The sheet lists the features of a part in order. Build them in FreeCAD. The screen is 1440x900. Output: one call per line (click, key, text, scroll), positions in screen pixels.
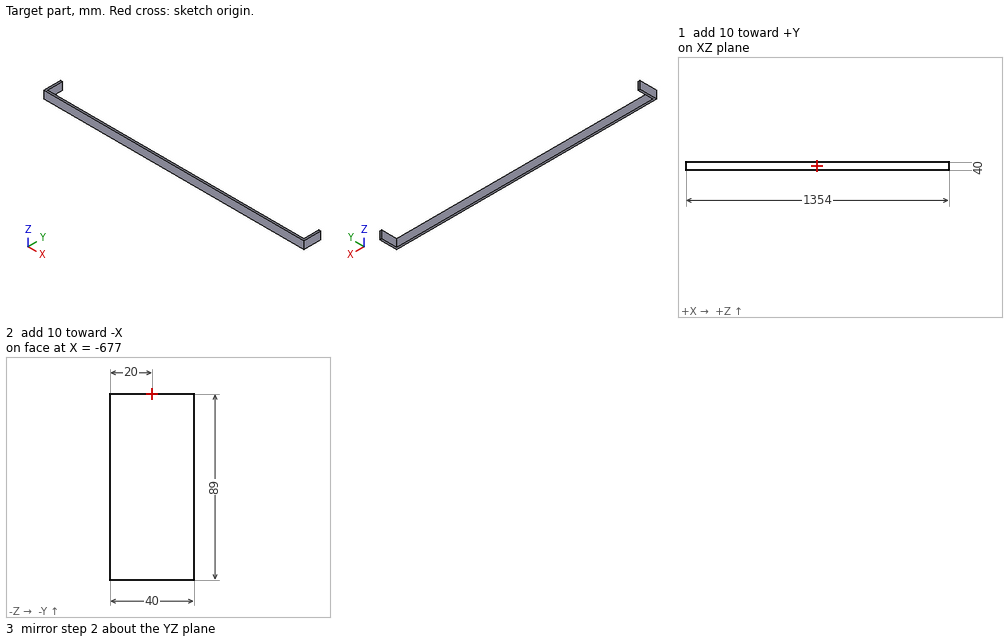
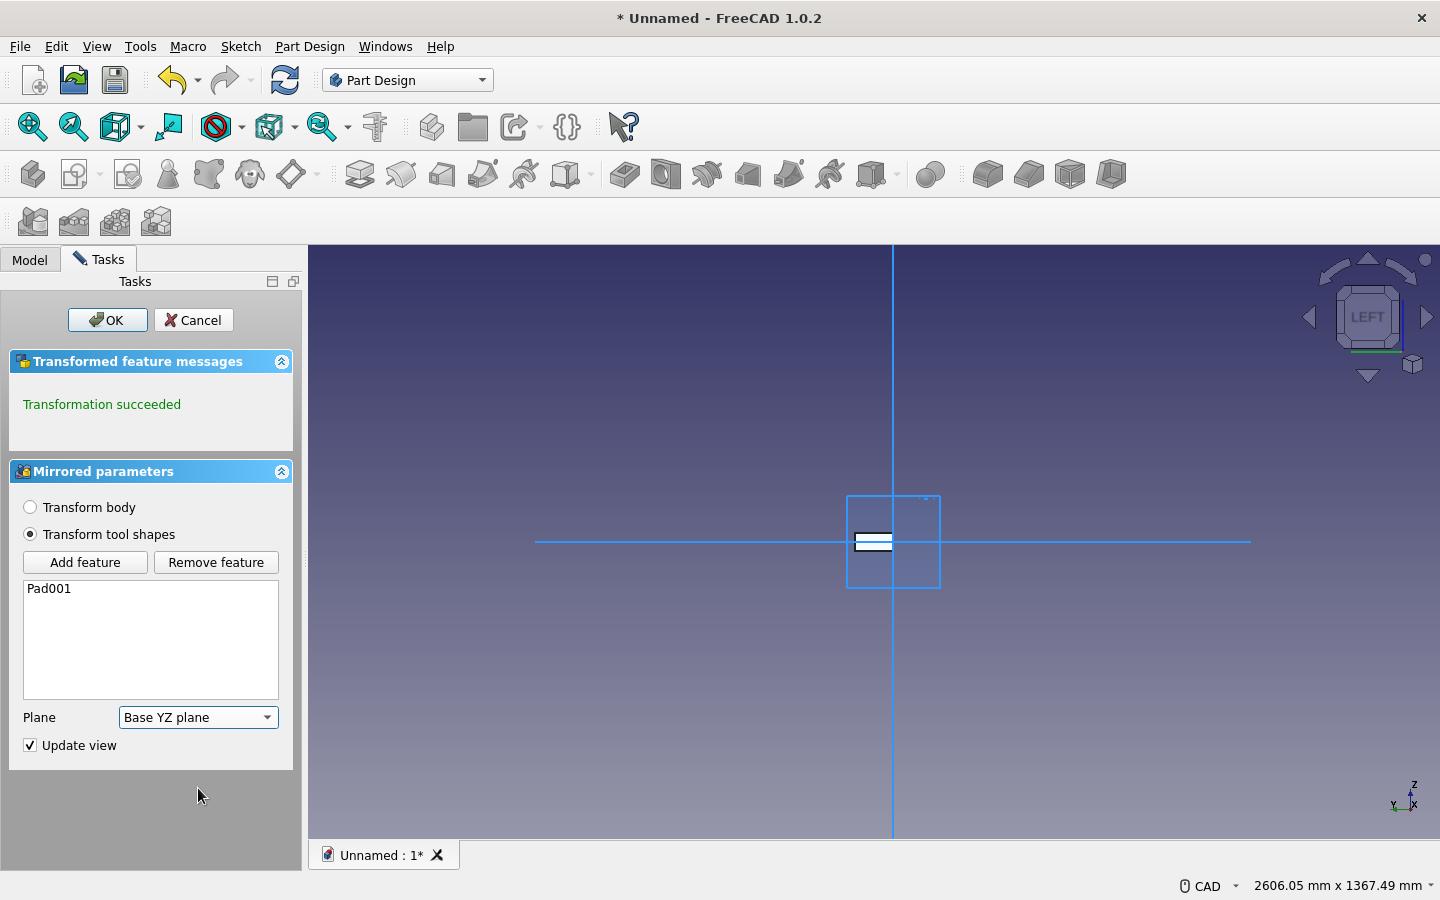
click(108, 320)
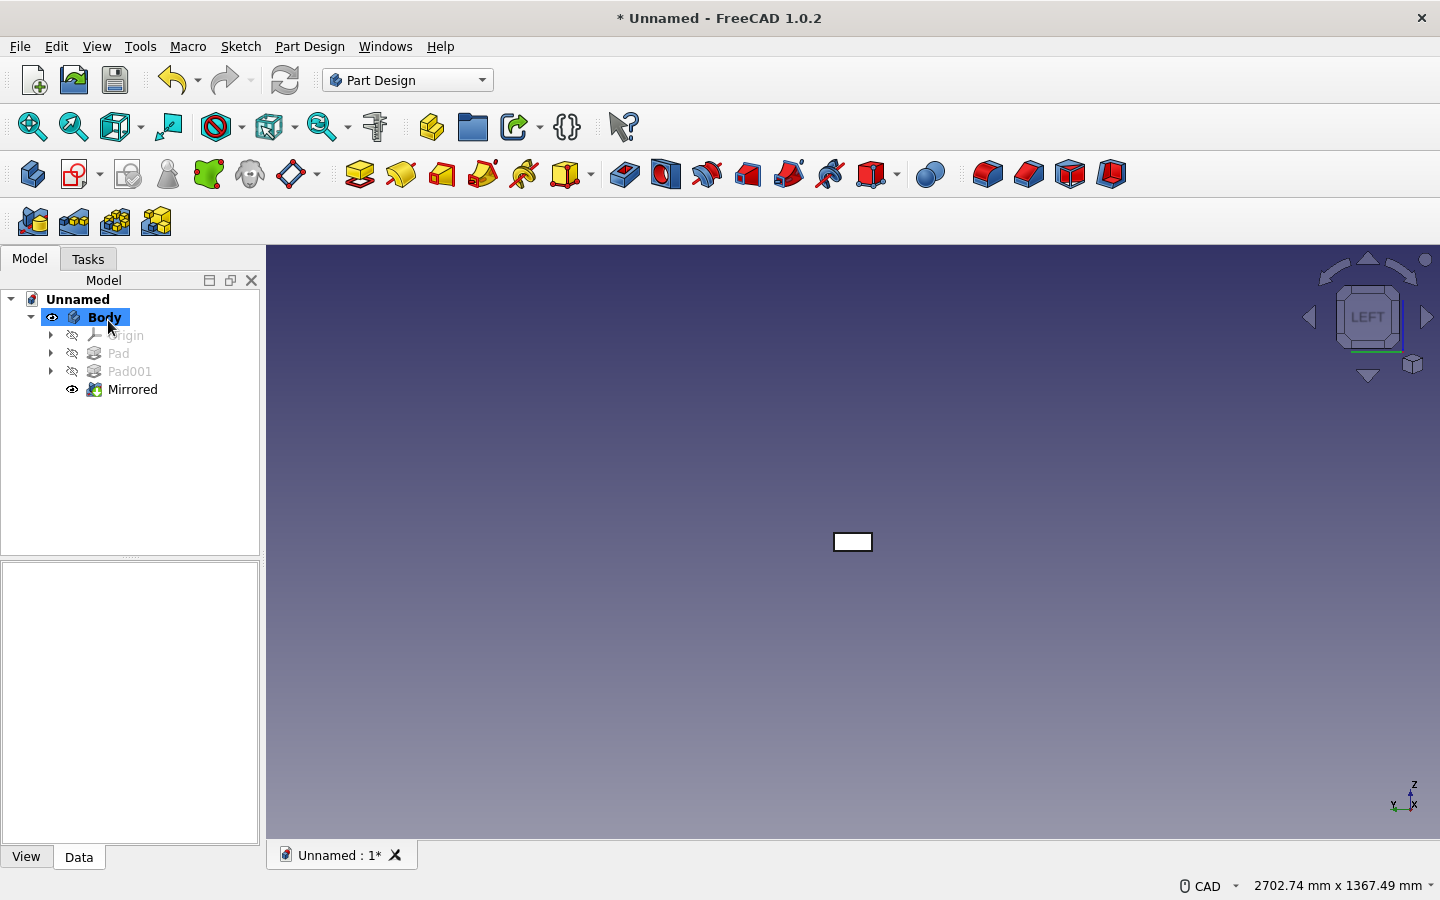
key(0)